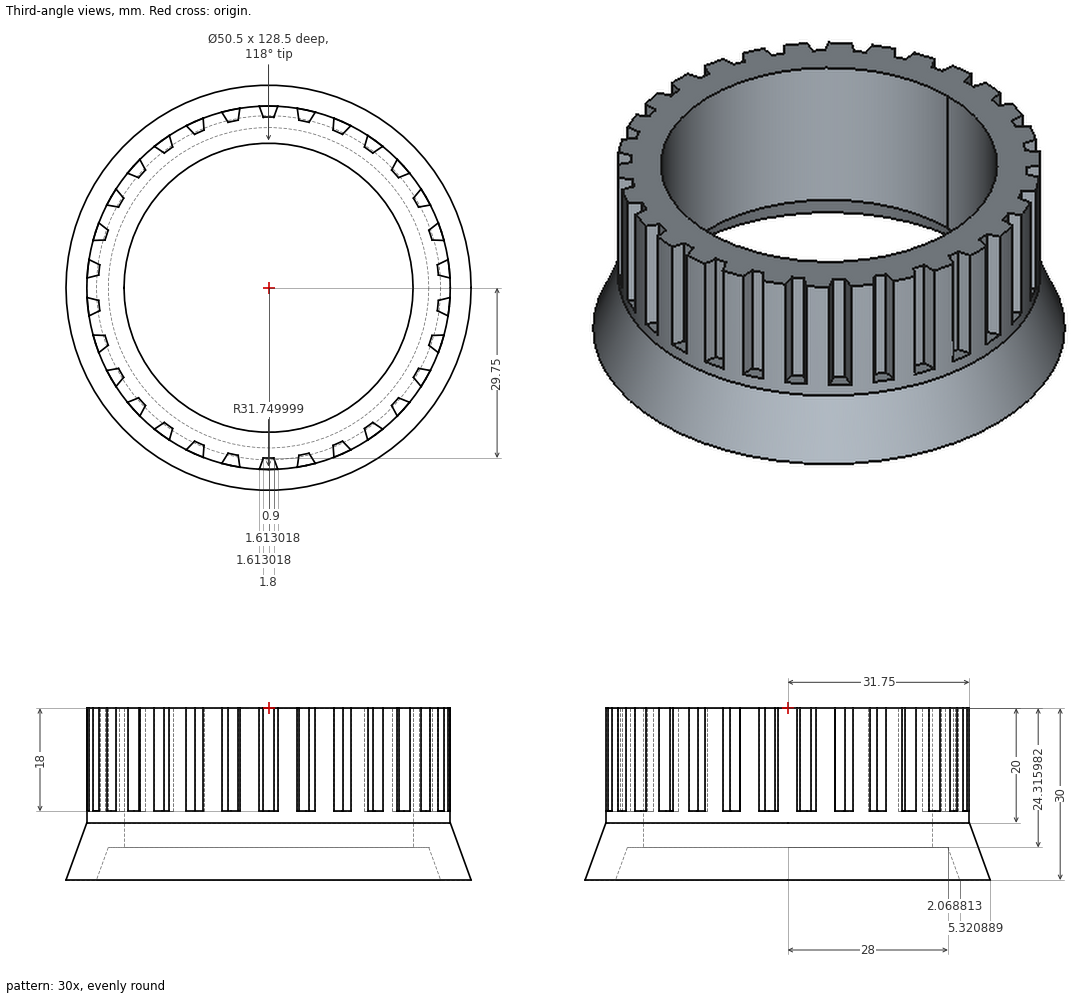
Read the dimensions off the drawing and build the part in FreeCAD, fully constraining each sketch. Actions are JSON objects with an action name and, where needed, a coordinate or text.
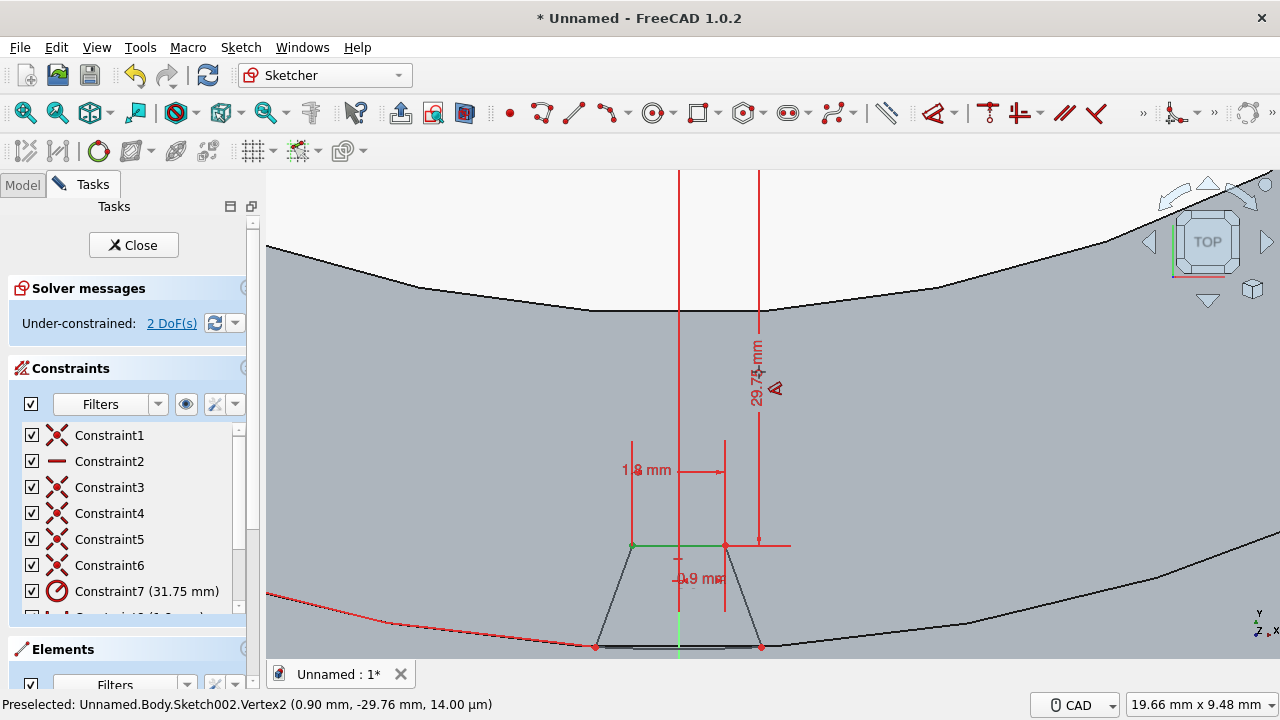
{"action": "scroll", "coordinate": [704, 414], "scroll_direction": "down", "scroll_amount": 5}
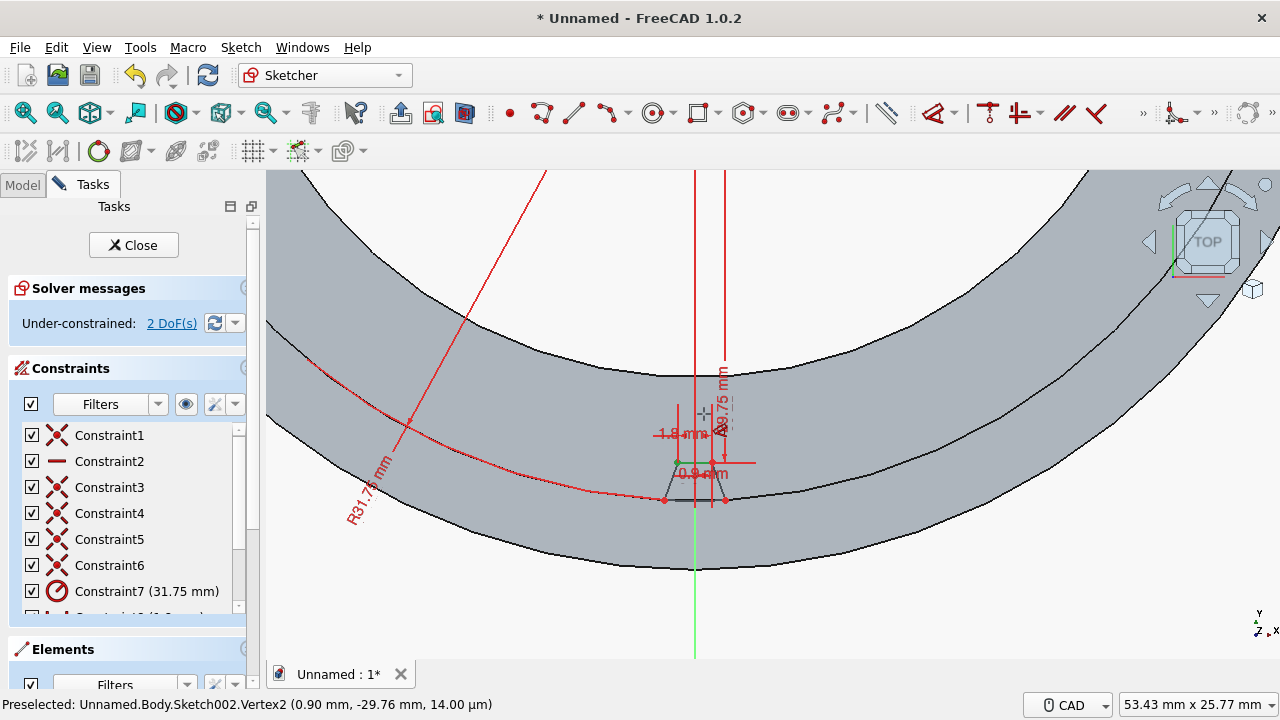
{"action": "scroll", "coordinate": [694, 492], "scroll_direction": "up", "scroll_amount": 10}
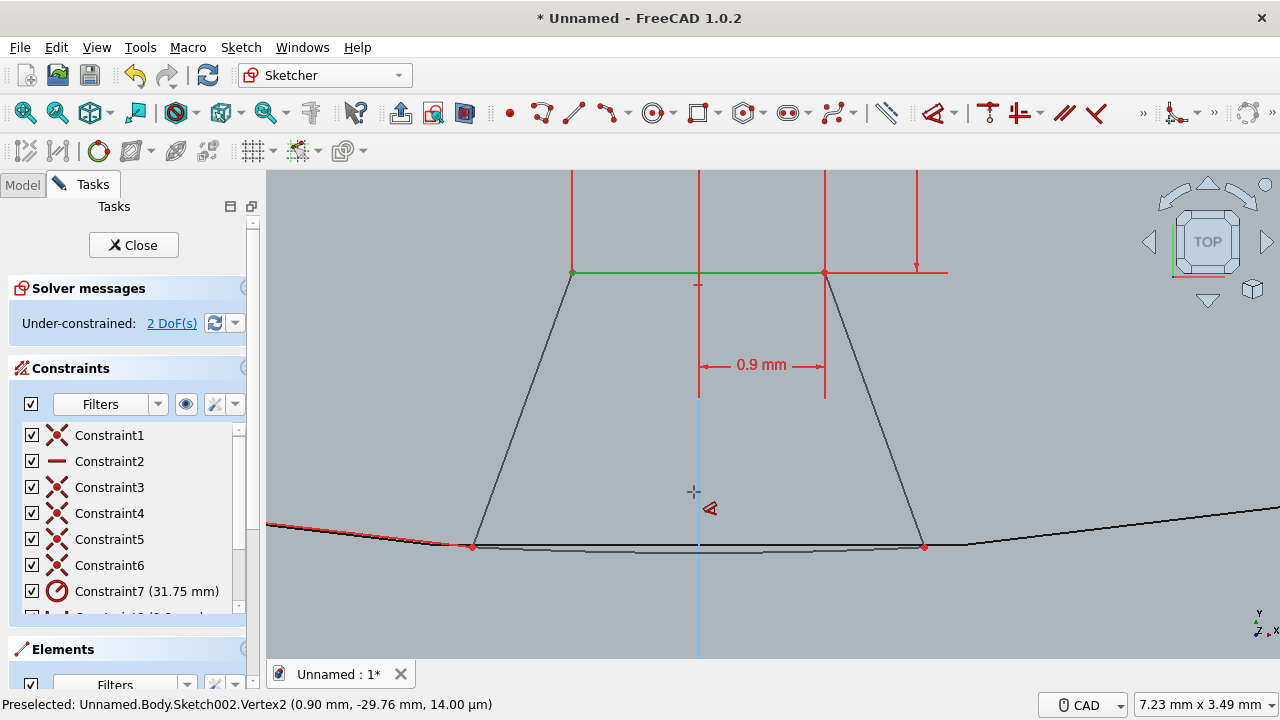
{"action": "left_click", "coordinate": [925, 547]}
{"action": "left_click", "coordinate": [812, 581]}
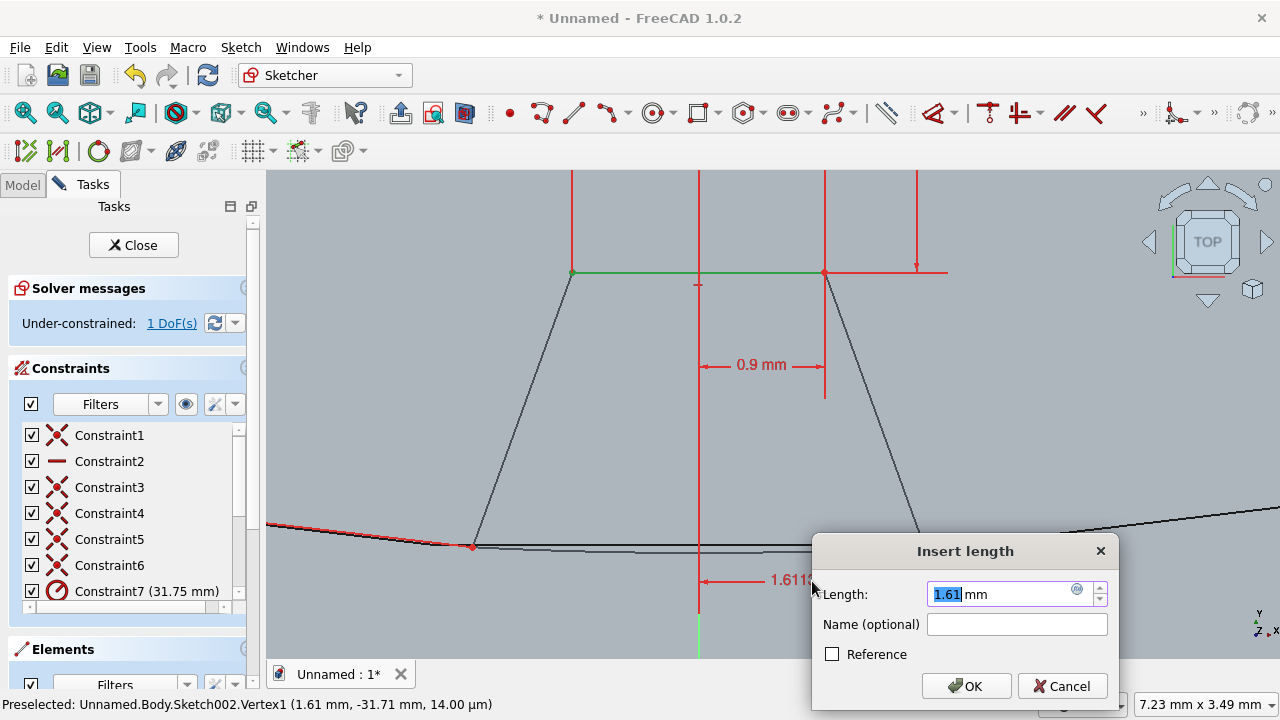
{"action": "type", "text": "1.613018"}
{"action": "key", "text": "Return"}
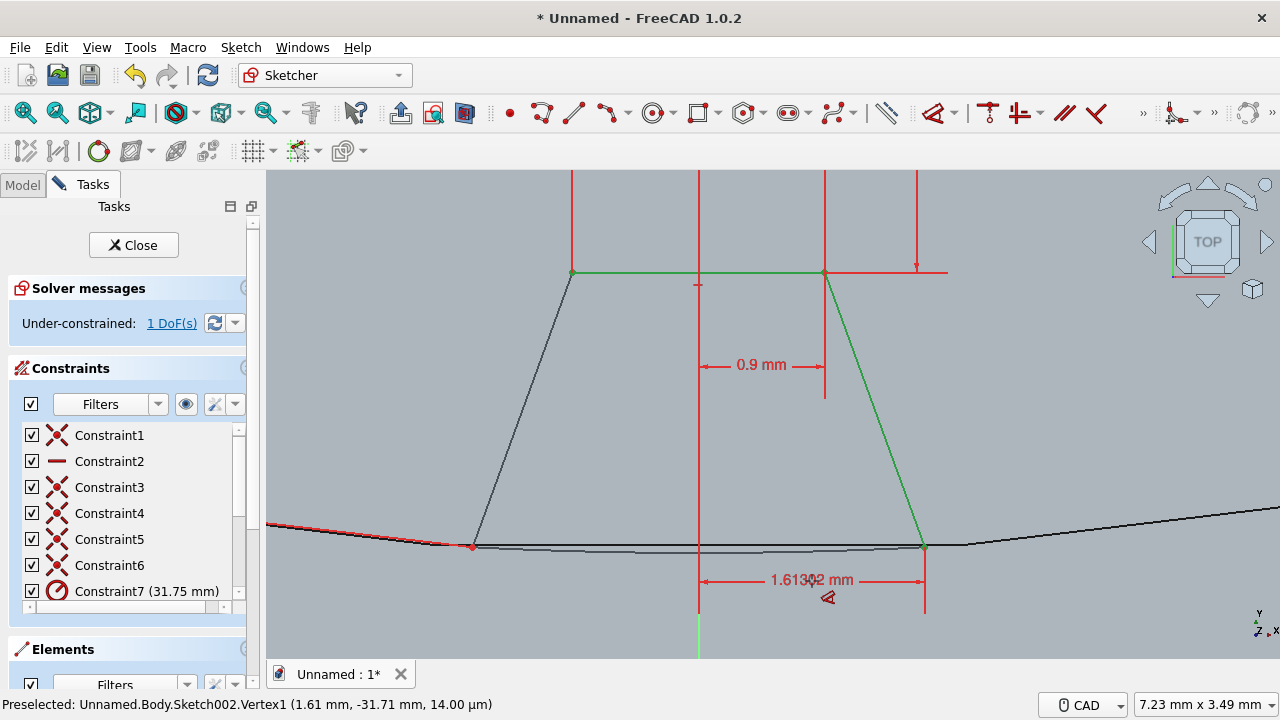
{"action": "left_click", "coordinate": [473, 547]}
{"action": "left_click", "coordinate": [586, 581]}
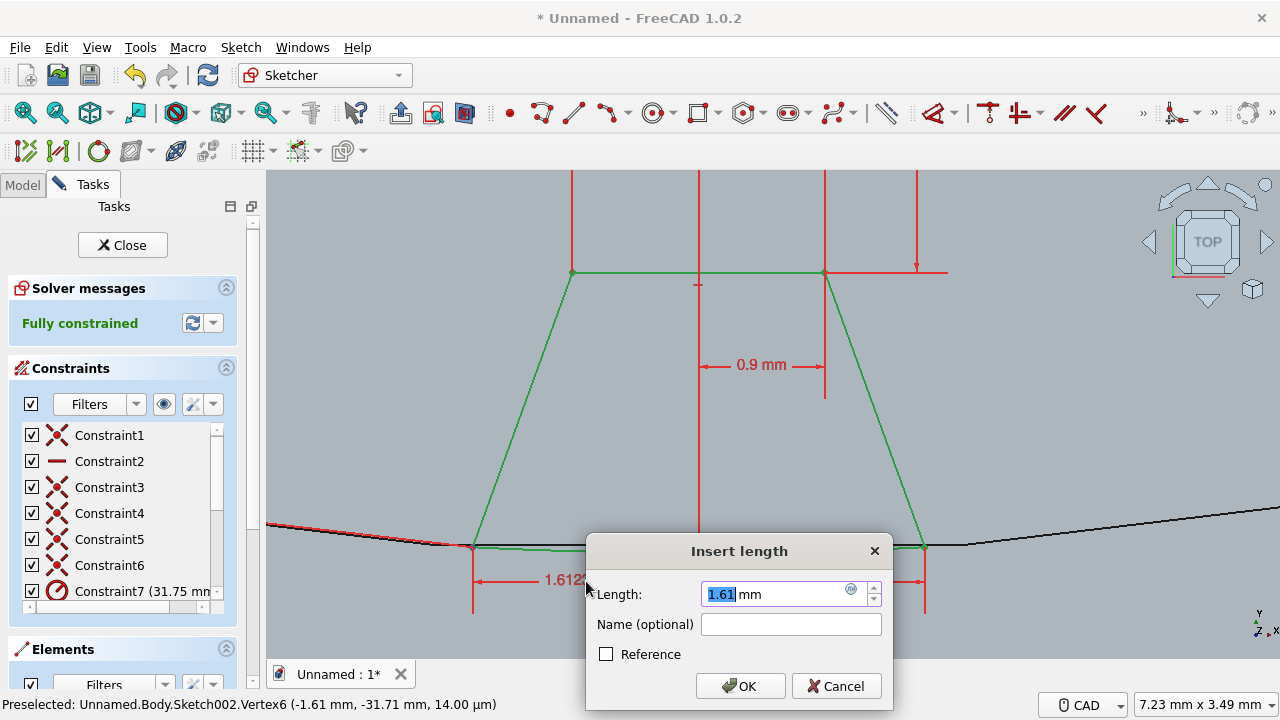
{"action": "type", "text": "1.613018"}
{"action": "key", "text": "Return"}
{"action": "key", "text": "Escape"}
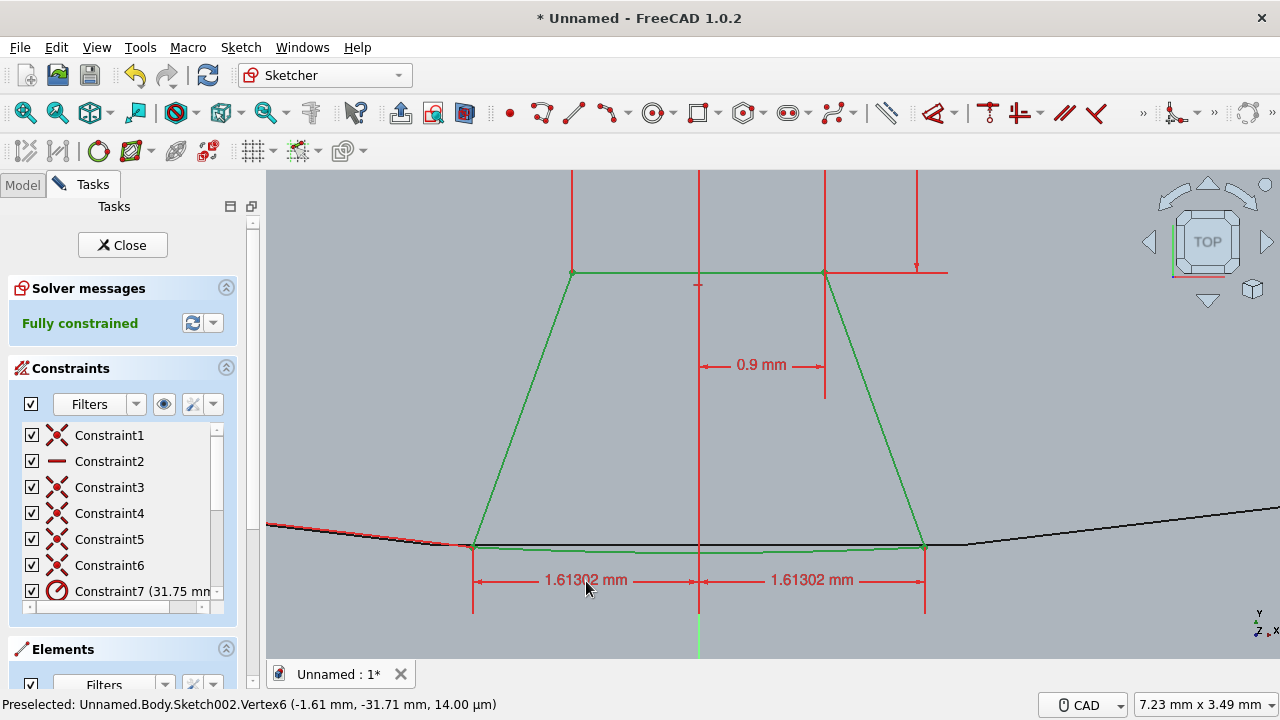
{"action": "left_click", "coordinate": [123, 245]}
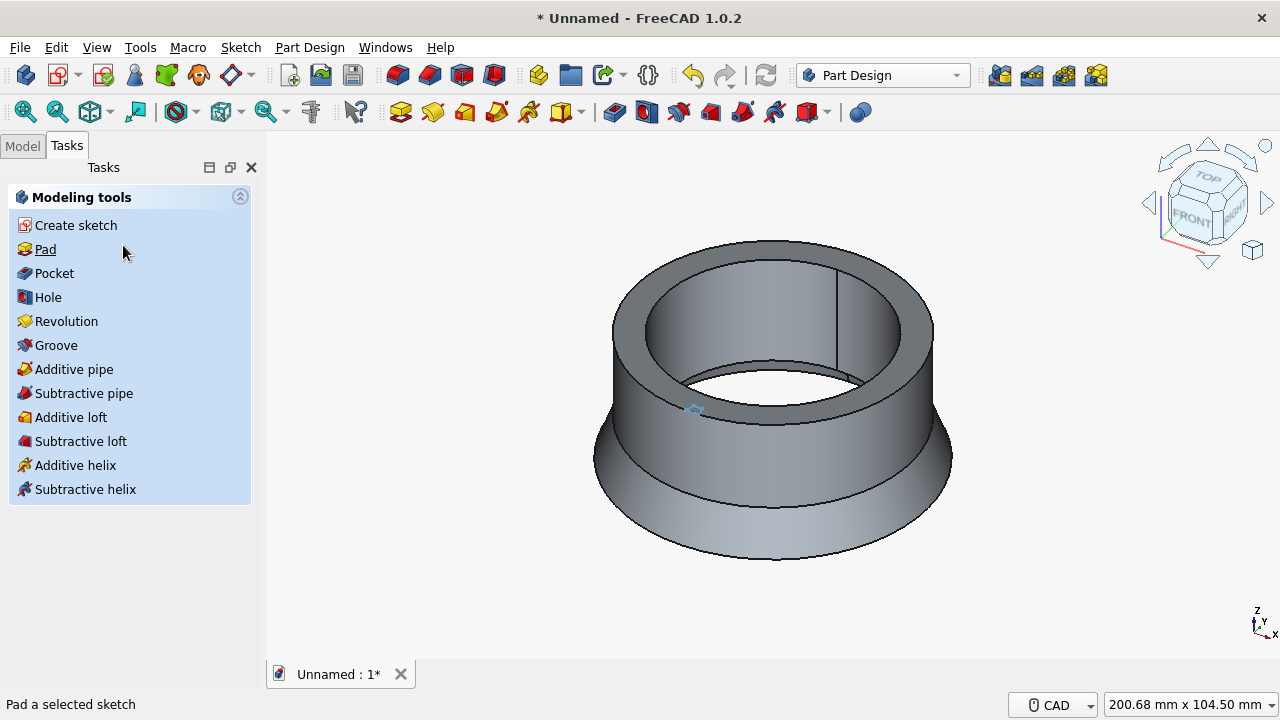
{"action": "left_click", "coordinate": [616, 112]}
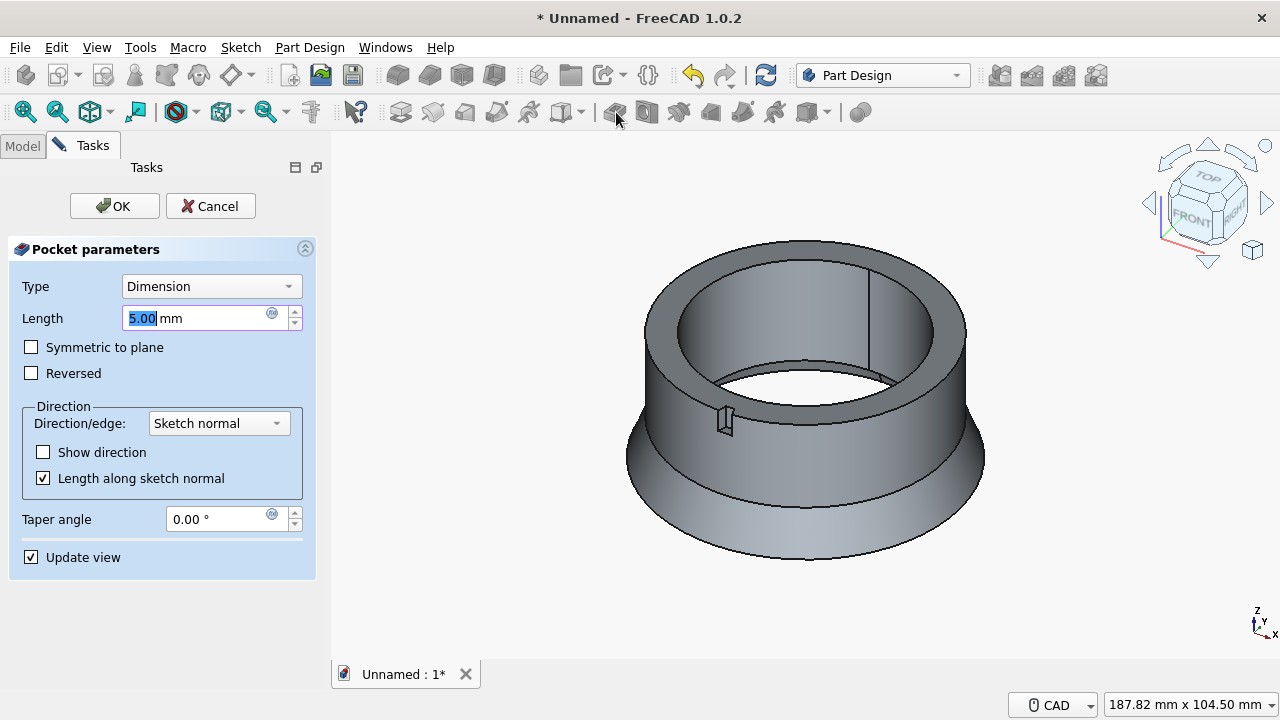
{"action": "type", "text": "18"}
{"action": "key", "text": "Tab"}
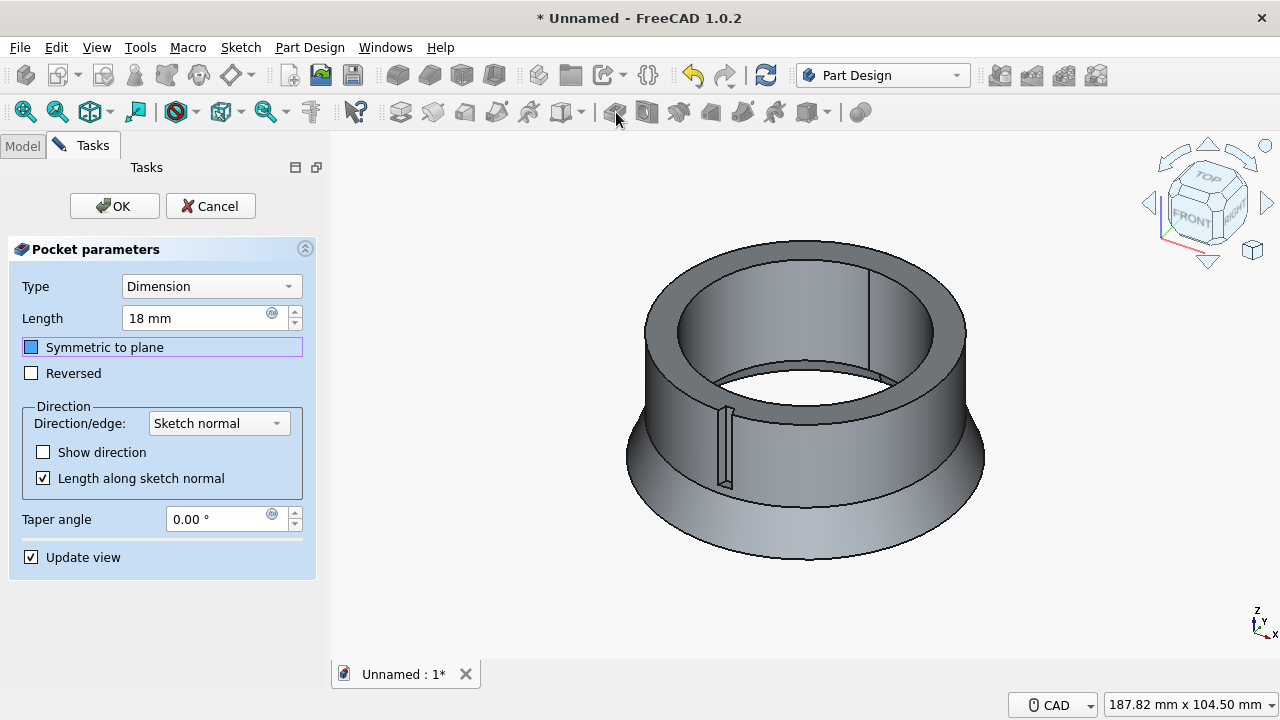
{"action": "left_click", "coordinate": [115, 206]}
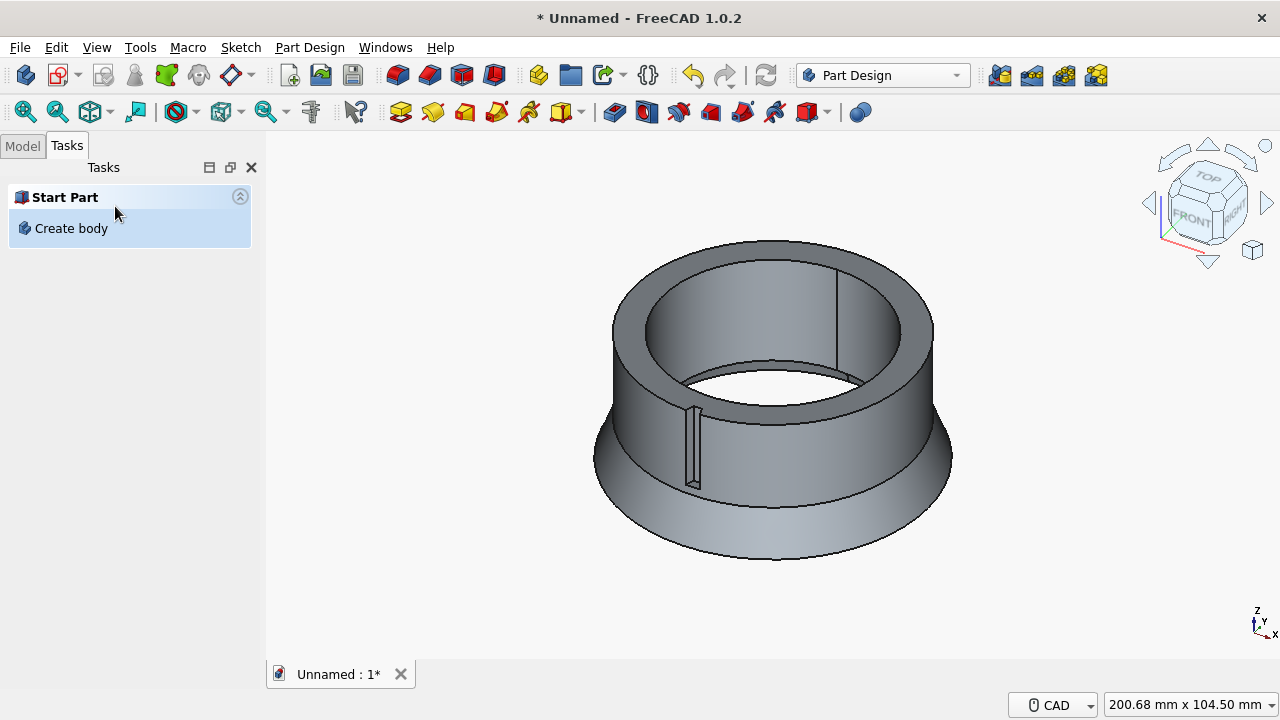
{"action": "left_click", "coordinate": [23, 145]}